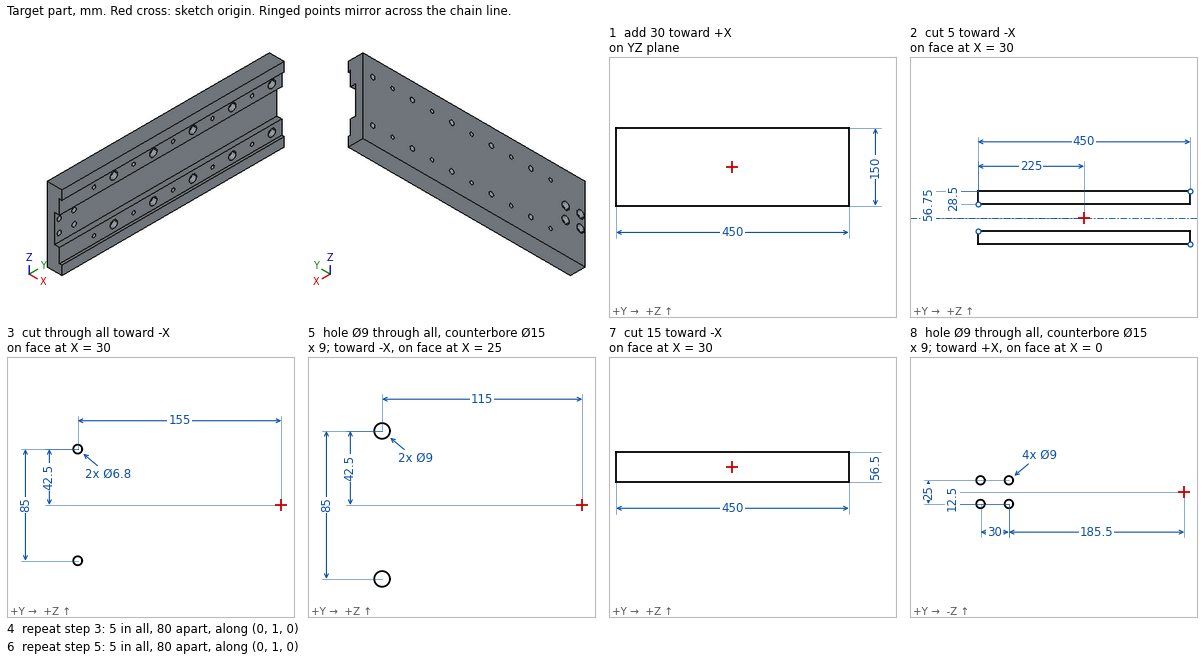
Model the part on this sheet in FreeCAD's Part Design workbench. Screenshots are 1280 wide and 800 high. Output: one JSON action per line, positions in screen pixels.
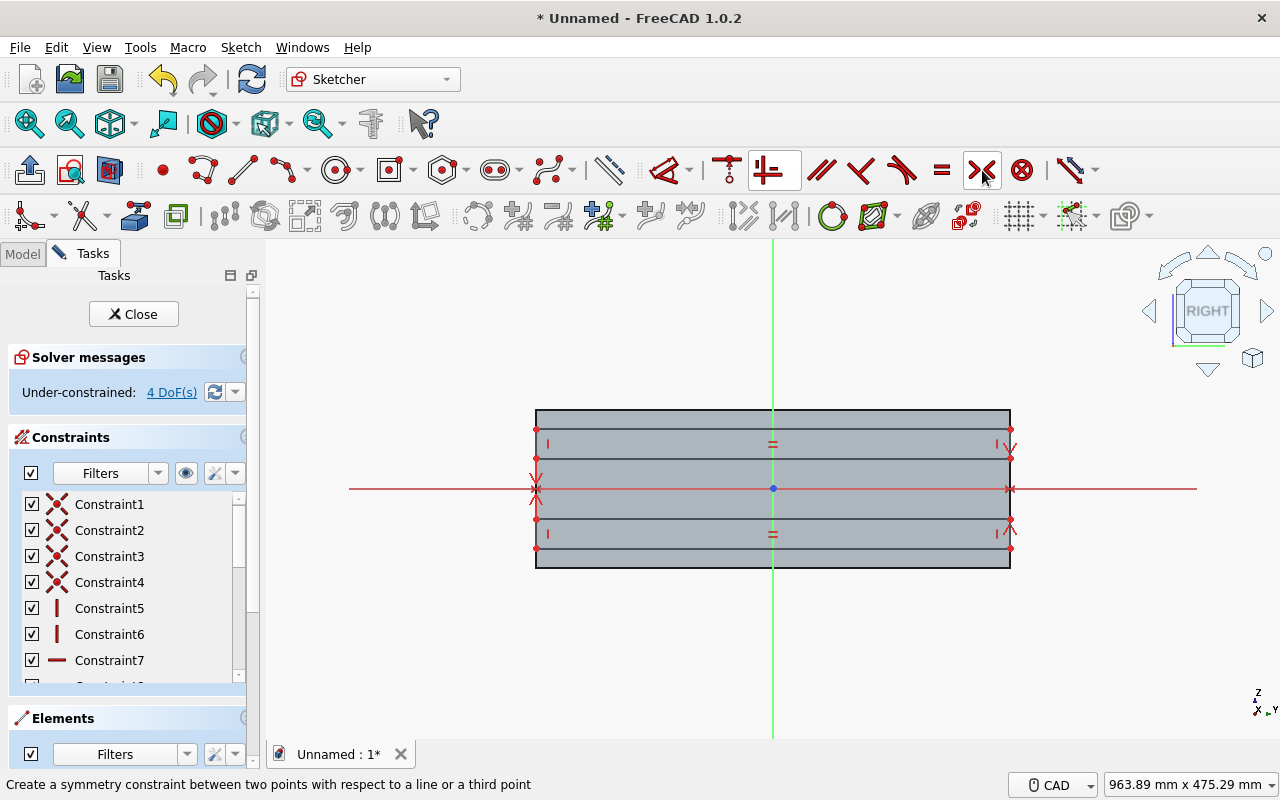
{"action": "left_click", "coordinate": [664, 170]}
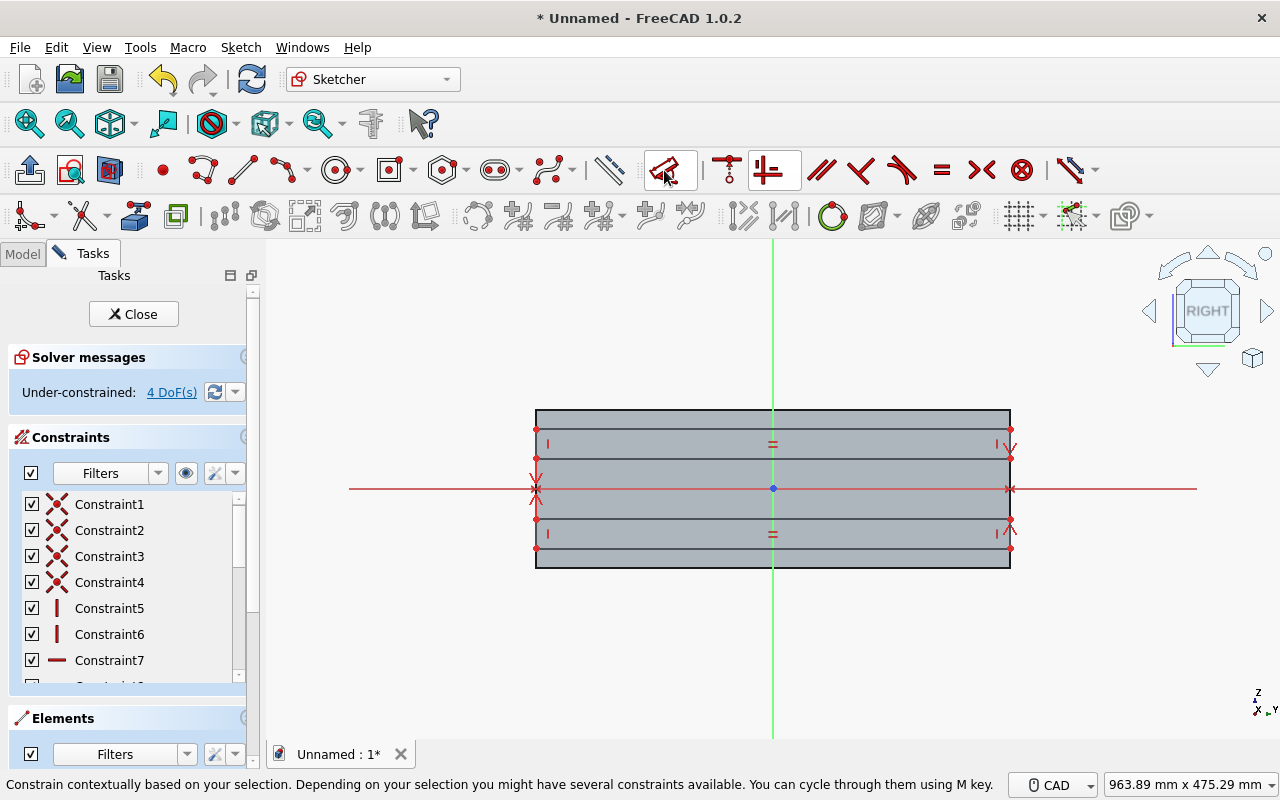
{"action": "left_click", "coordinate": [678, 459]}
{"action": "left_click", "coordinate": [664, 401]}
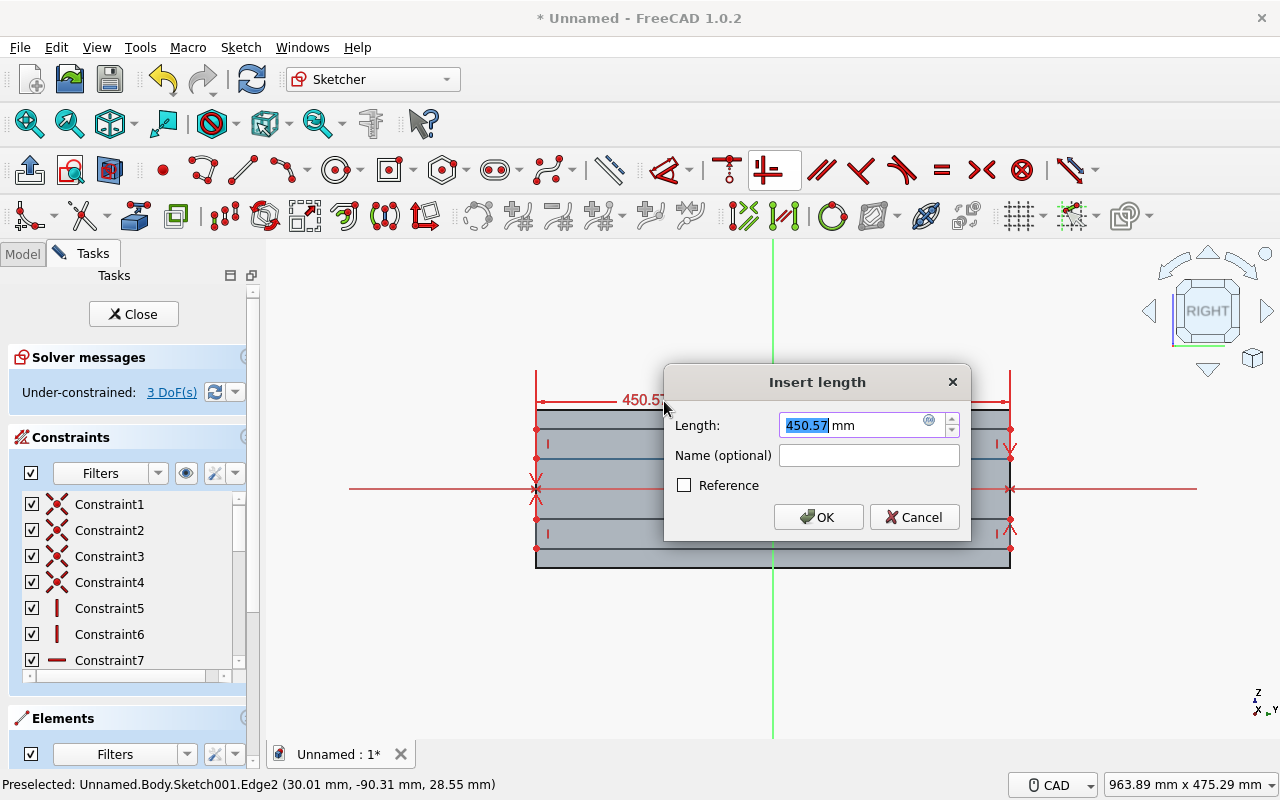
{"action": "type", "text": "450"}
{"action": "key", "text": "Return"}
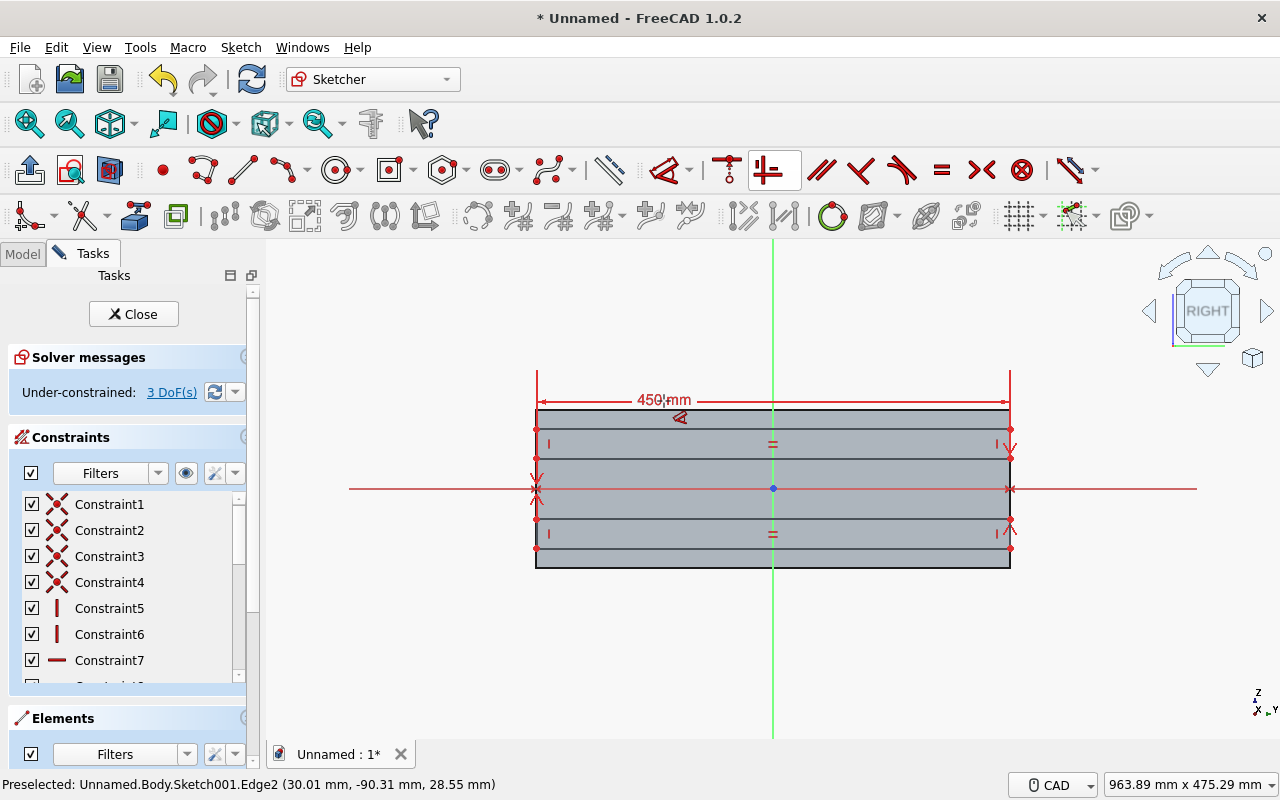
{"action": "scroll", "coordinate": [537, 441], "scroll_direction": "up", "scroll_amount": 2}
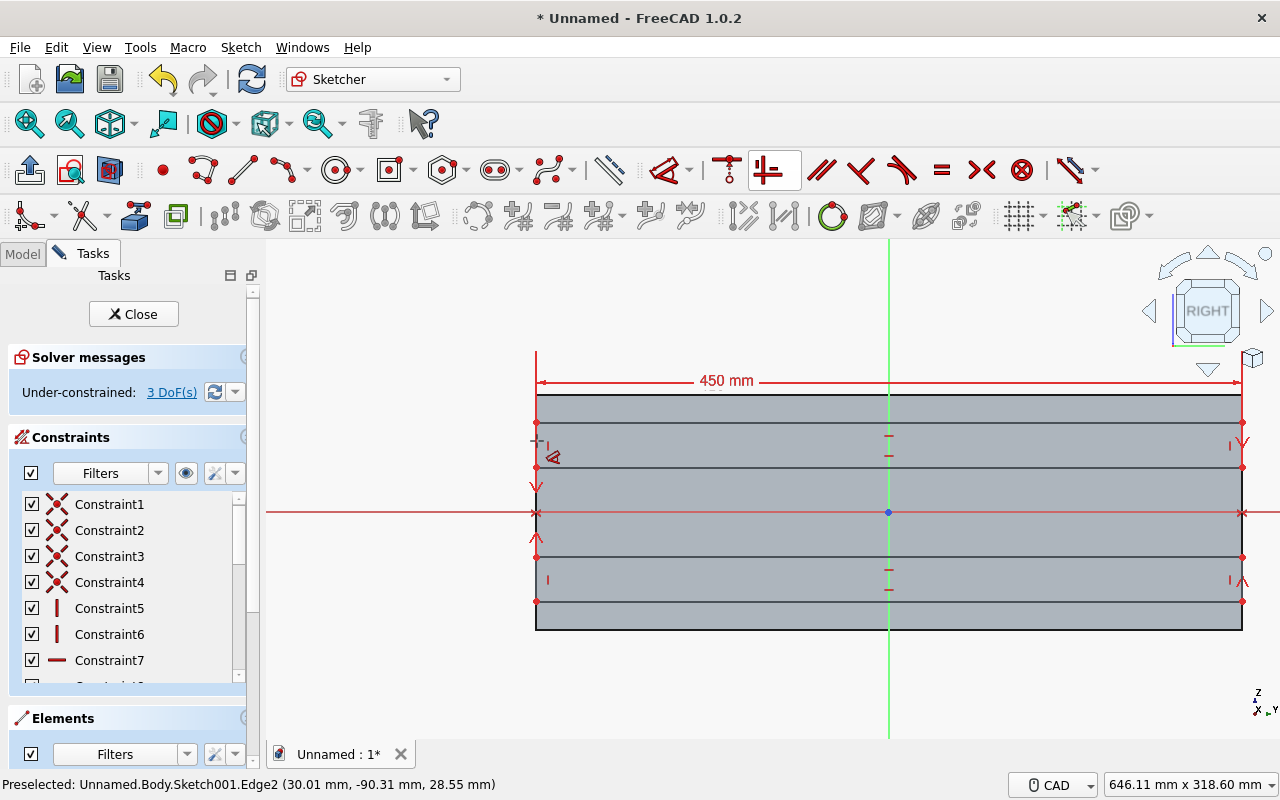
{"action": "left_click", "coordinate": [536, 441]}
{"action": "left_click", "coordinate": [502, 445]}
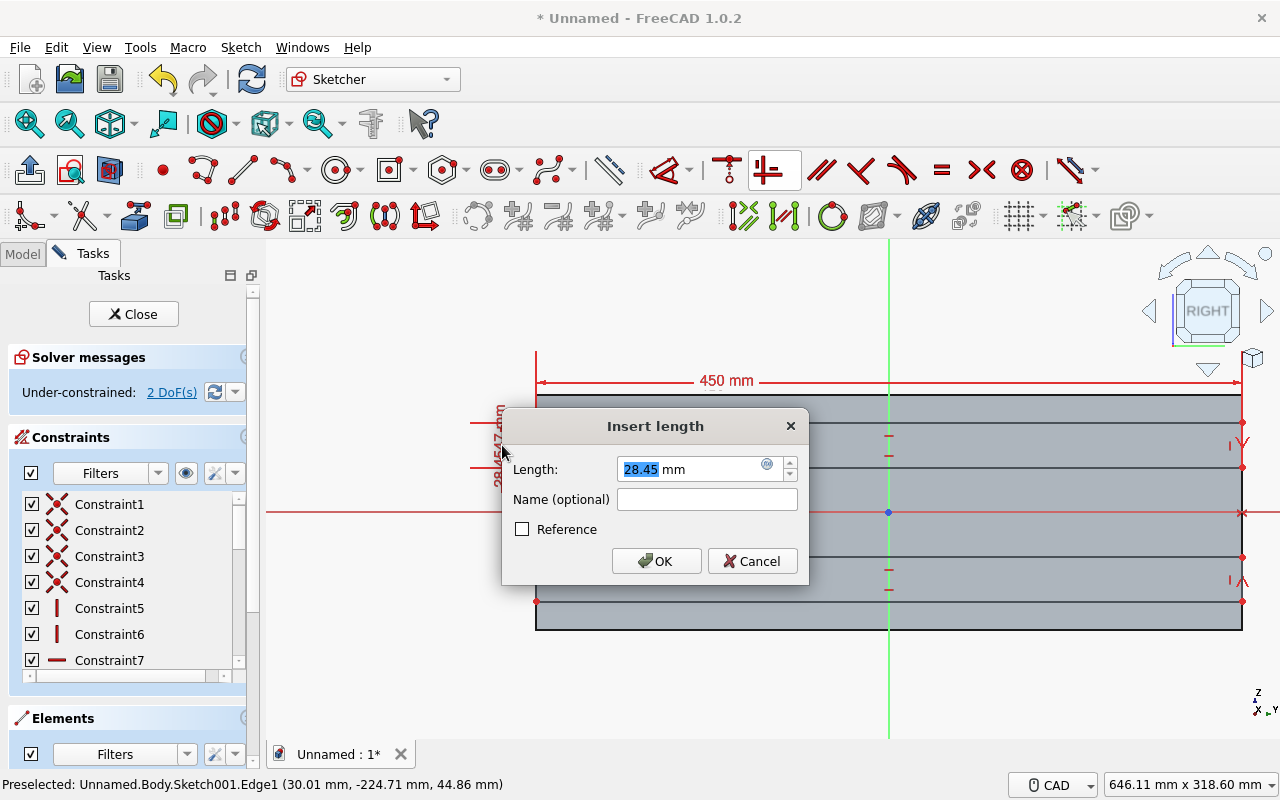
{"action": "type", "text": "28.5"}
{"action": "key", "text": "Return"}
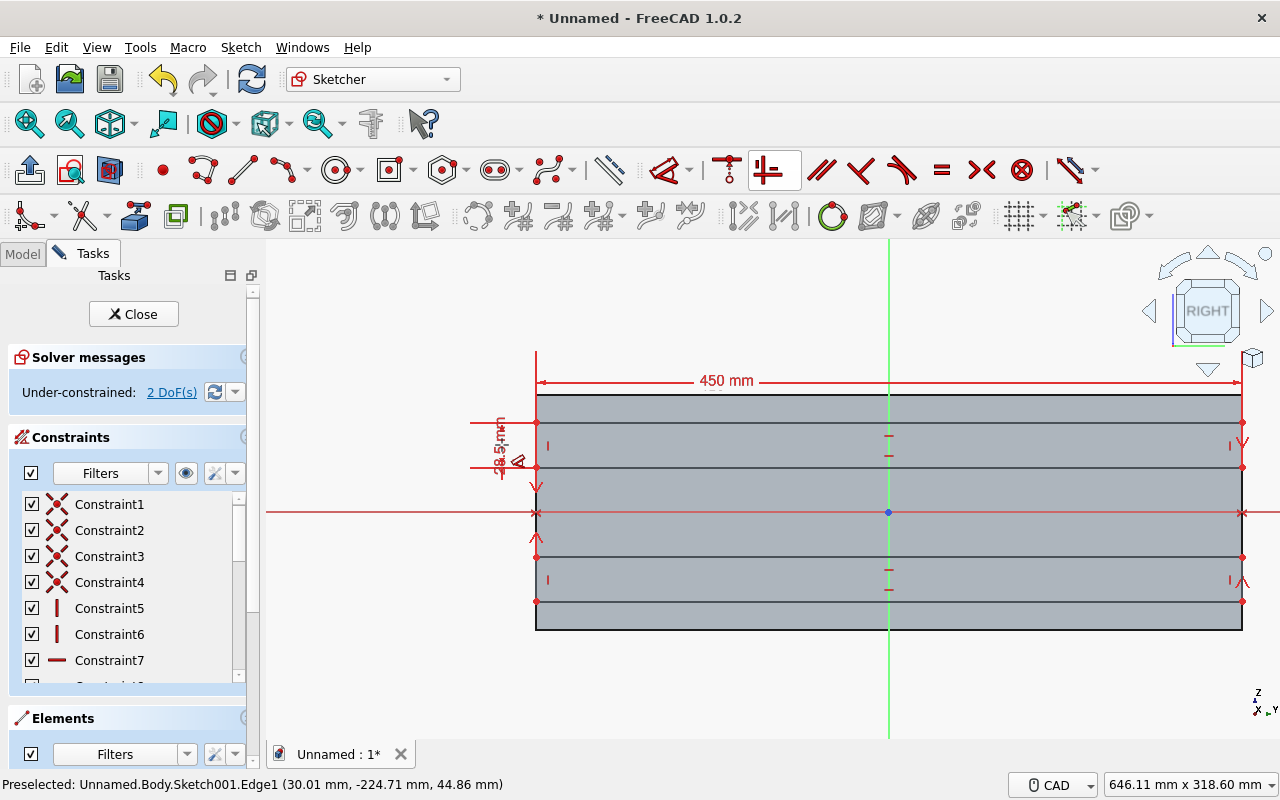
{"action": "left_click", "coordinate": [536, 423]}
{"action": "left_click", "coordinate": [631, 389]}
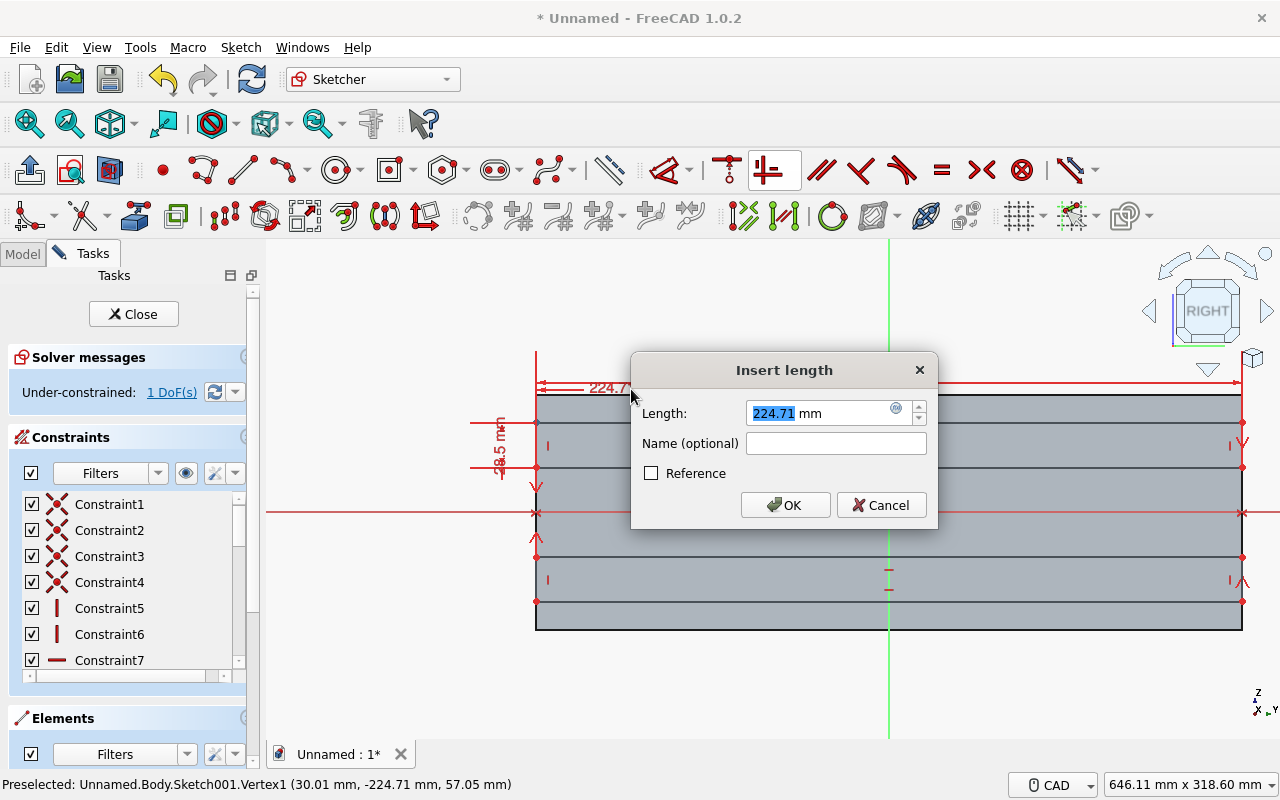
{"action": "type", "text": "225"}
{"action": "key", "text": "Return"}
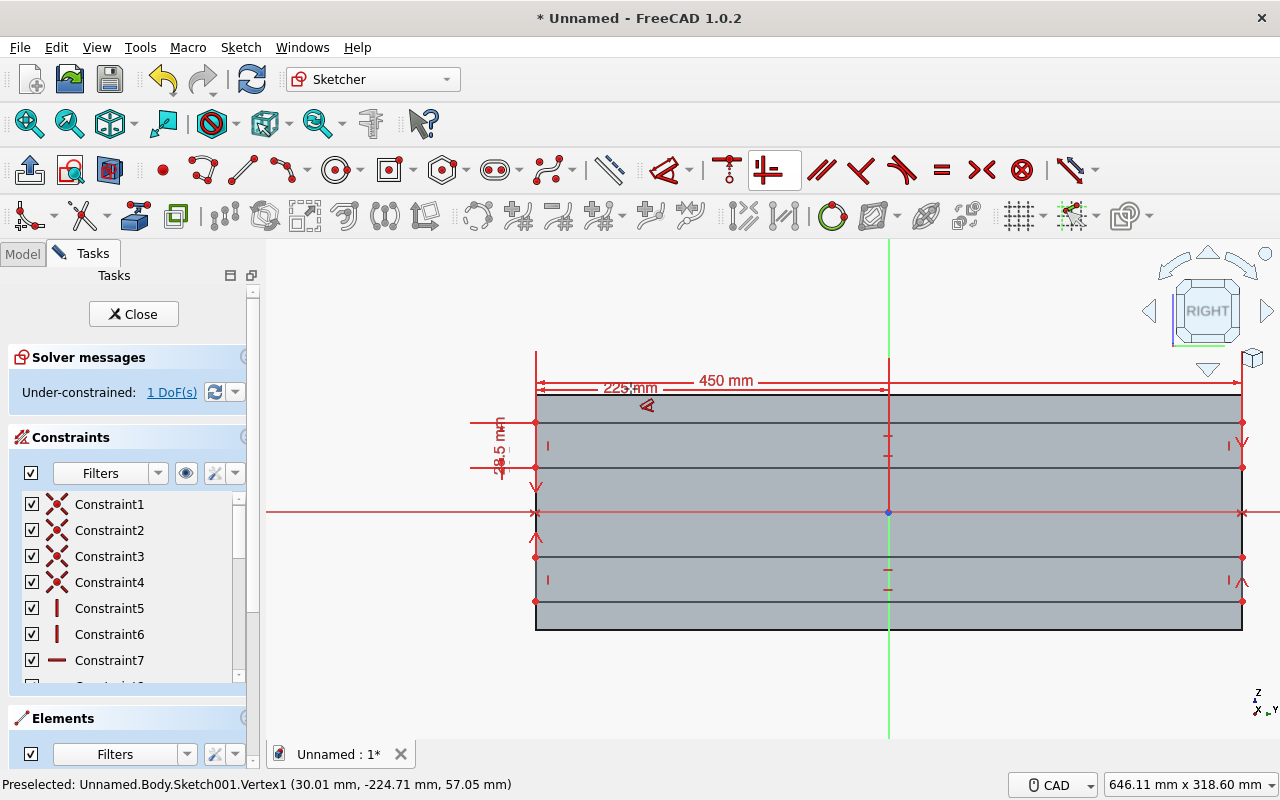
{"action": "left_click", "coordinate": [536, 423]}
{"action": "left_click", "coordinate": [502, 468]}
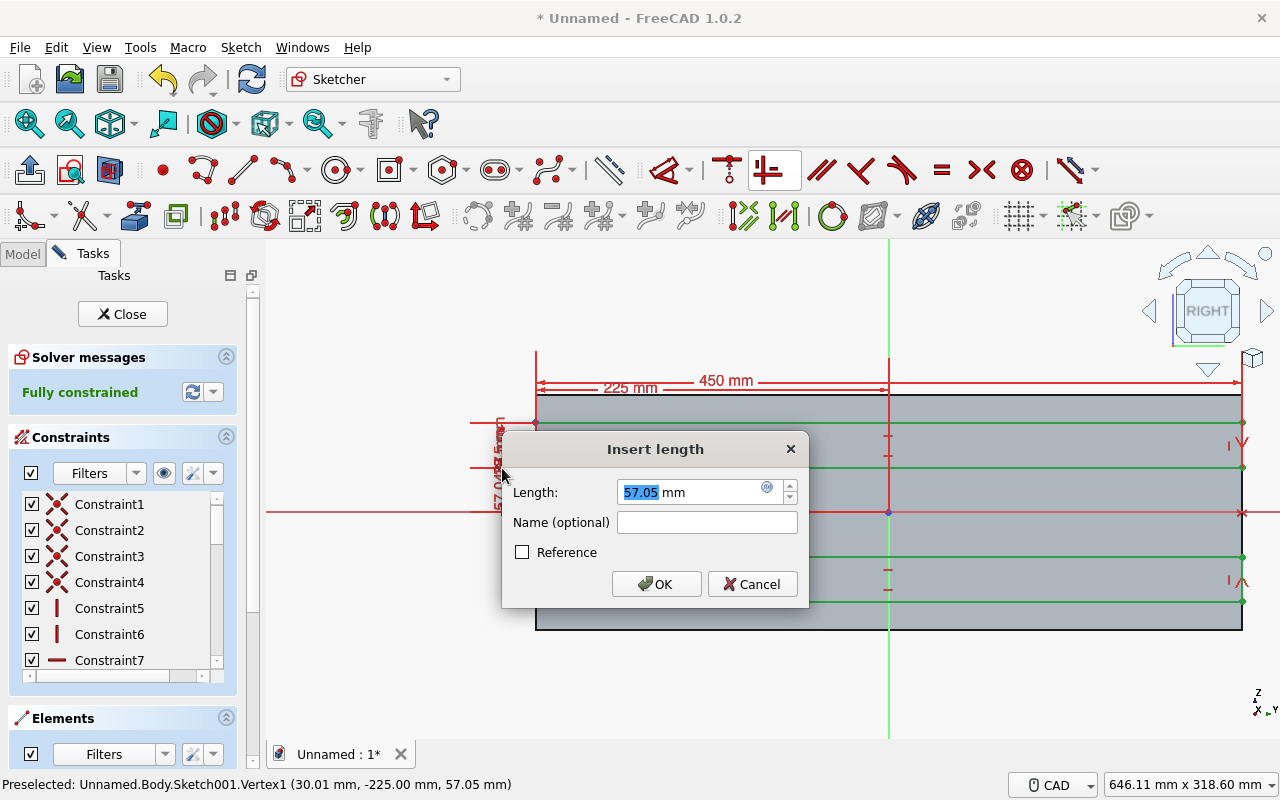
{"action": "type", "text": "56.75"}
{"action": "key", "text": "Return"}
{"action": "key", "text": "Escape"}